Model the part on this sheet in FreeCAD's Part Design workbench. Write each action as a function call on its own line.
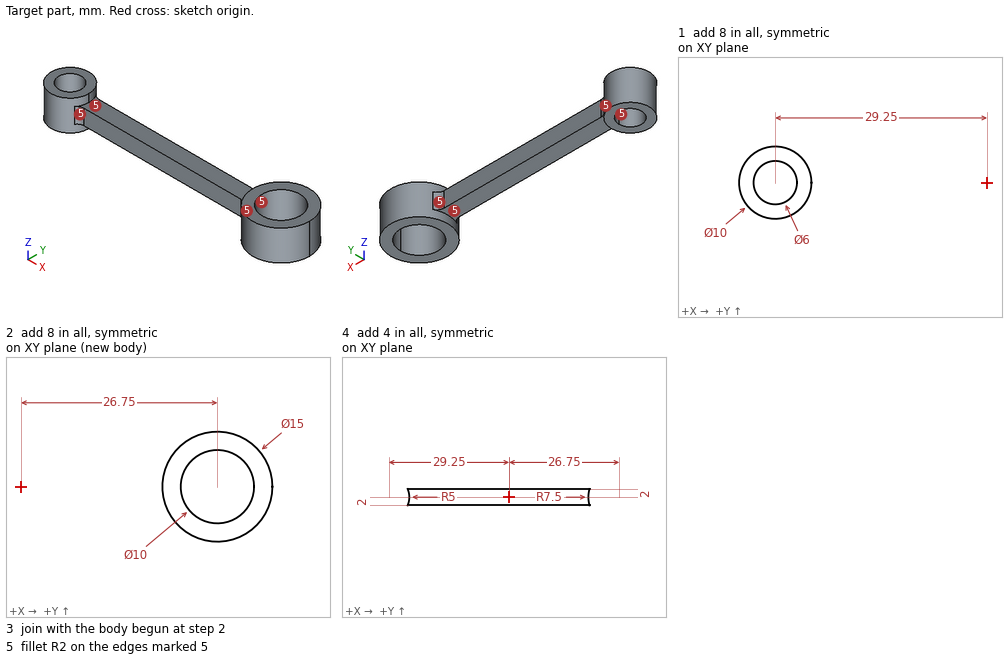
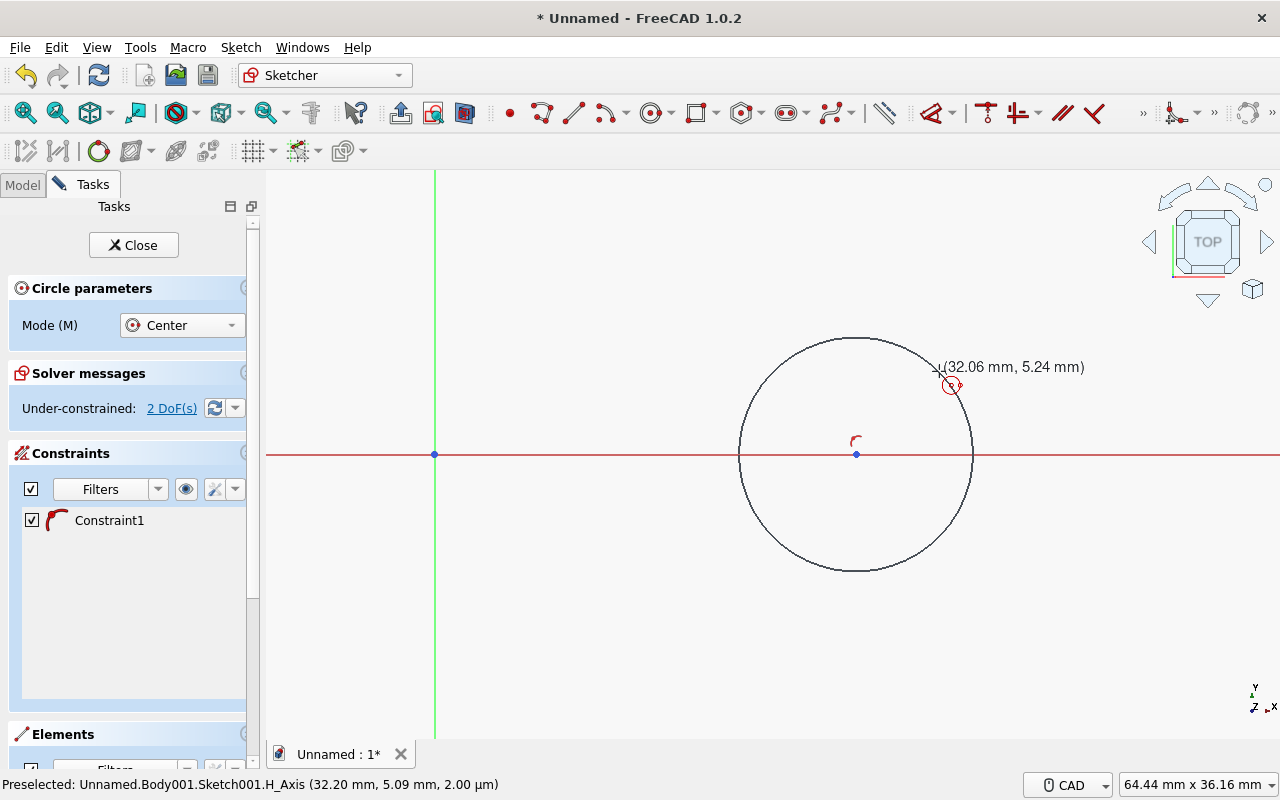
click(856, 454)
click(911, 399)
key(Escape)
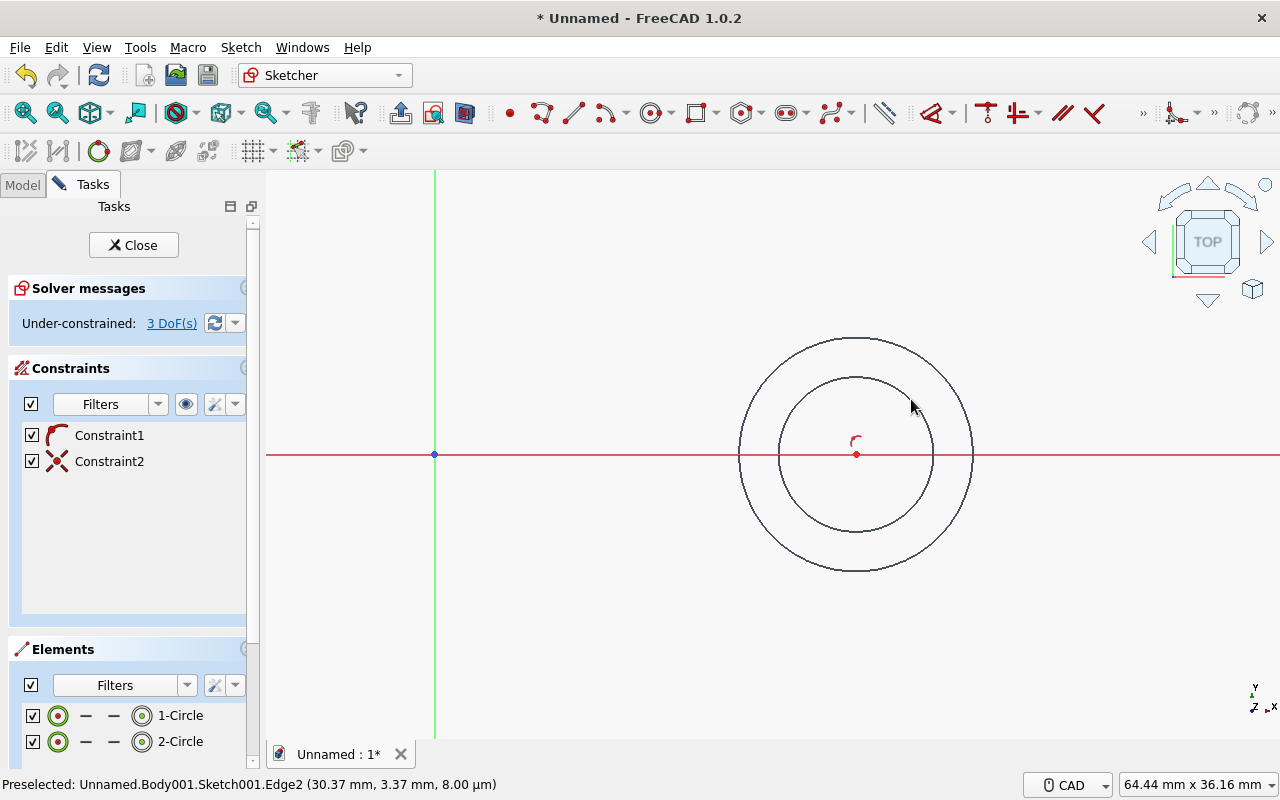
click(932, 114)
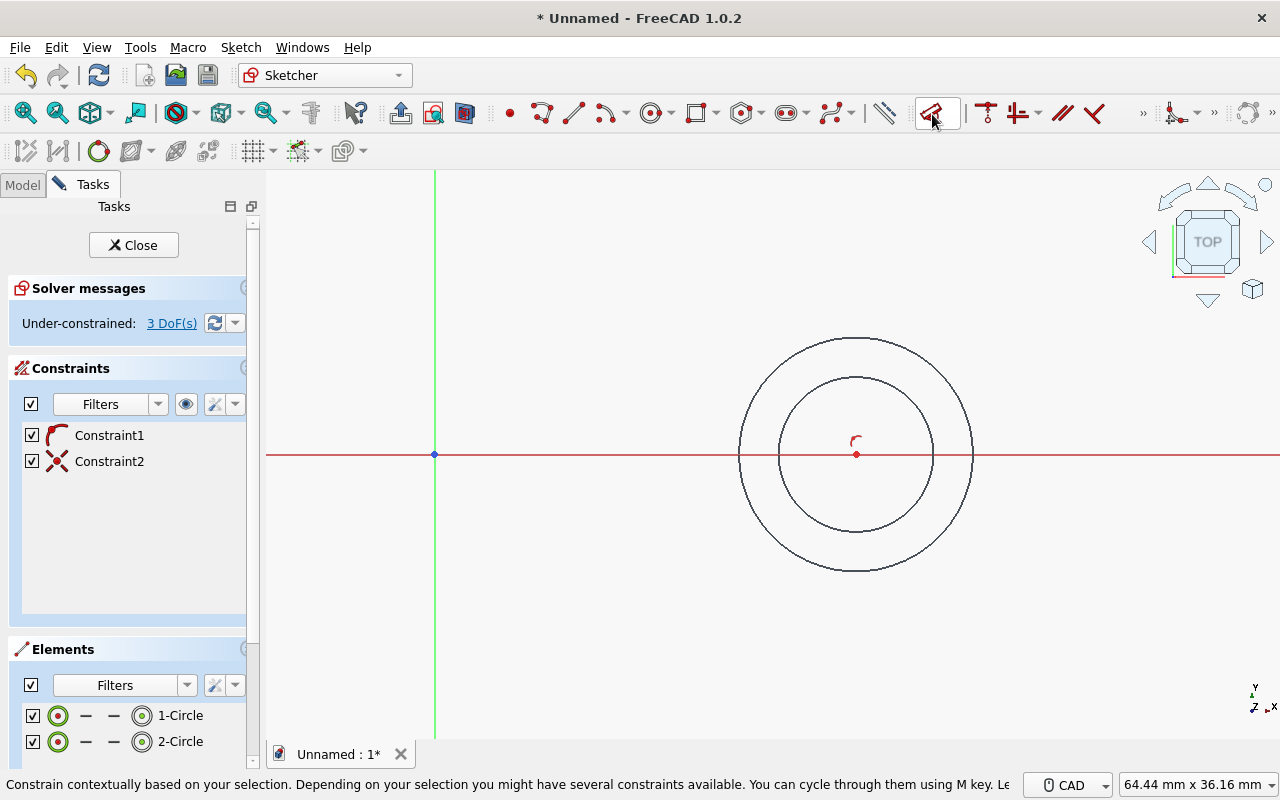
click(938, 371)
click(960, 348)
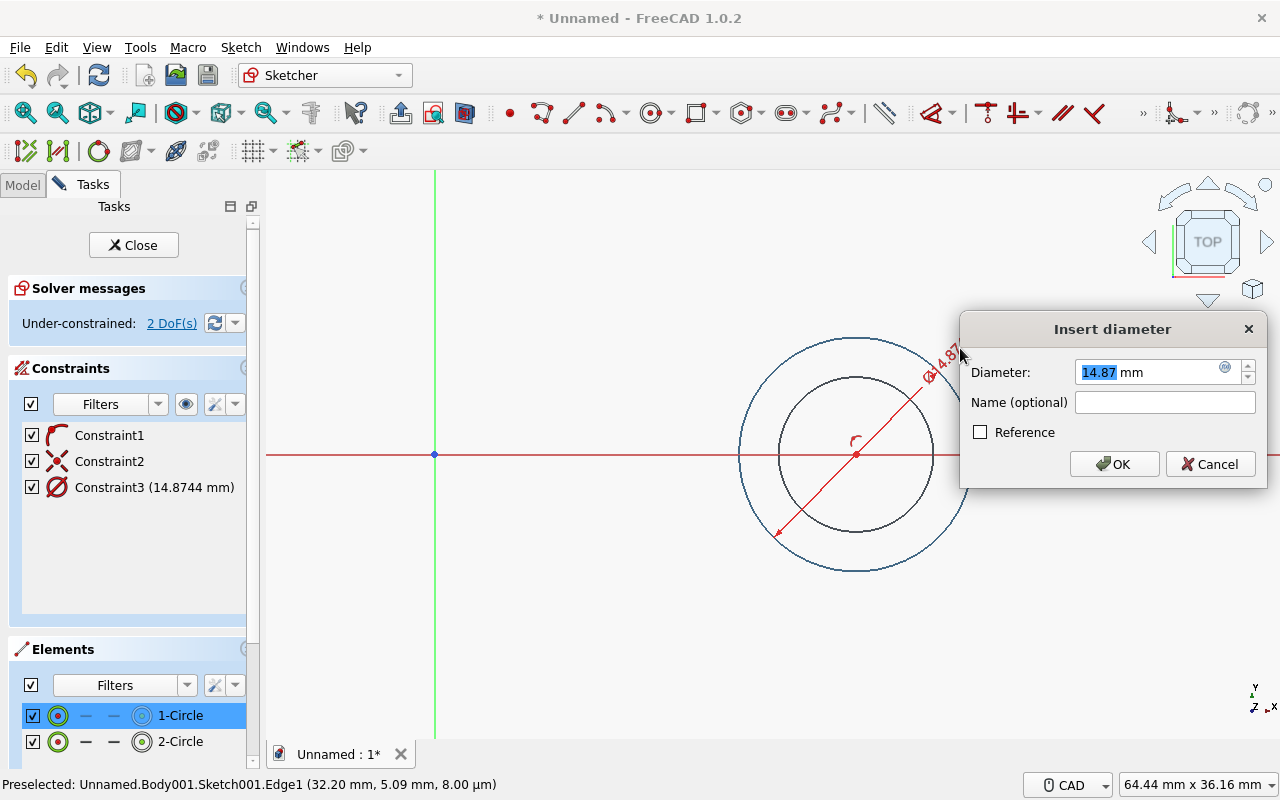
text(15)
key(Return)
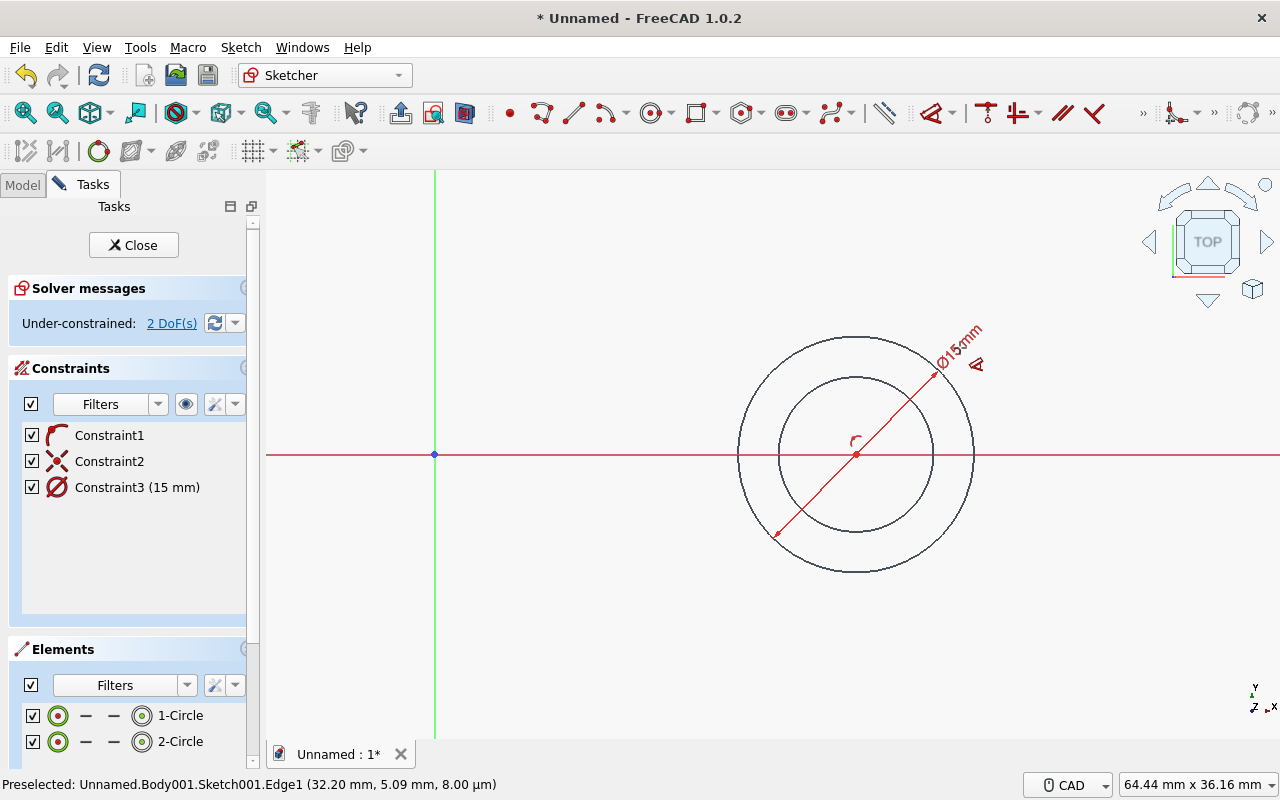
click(911, 400)
click(983, 418)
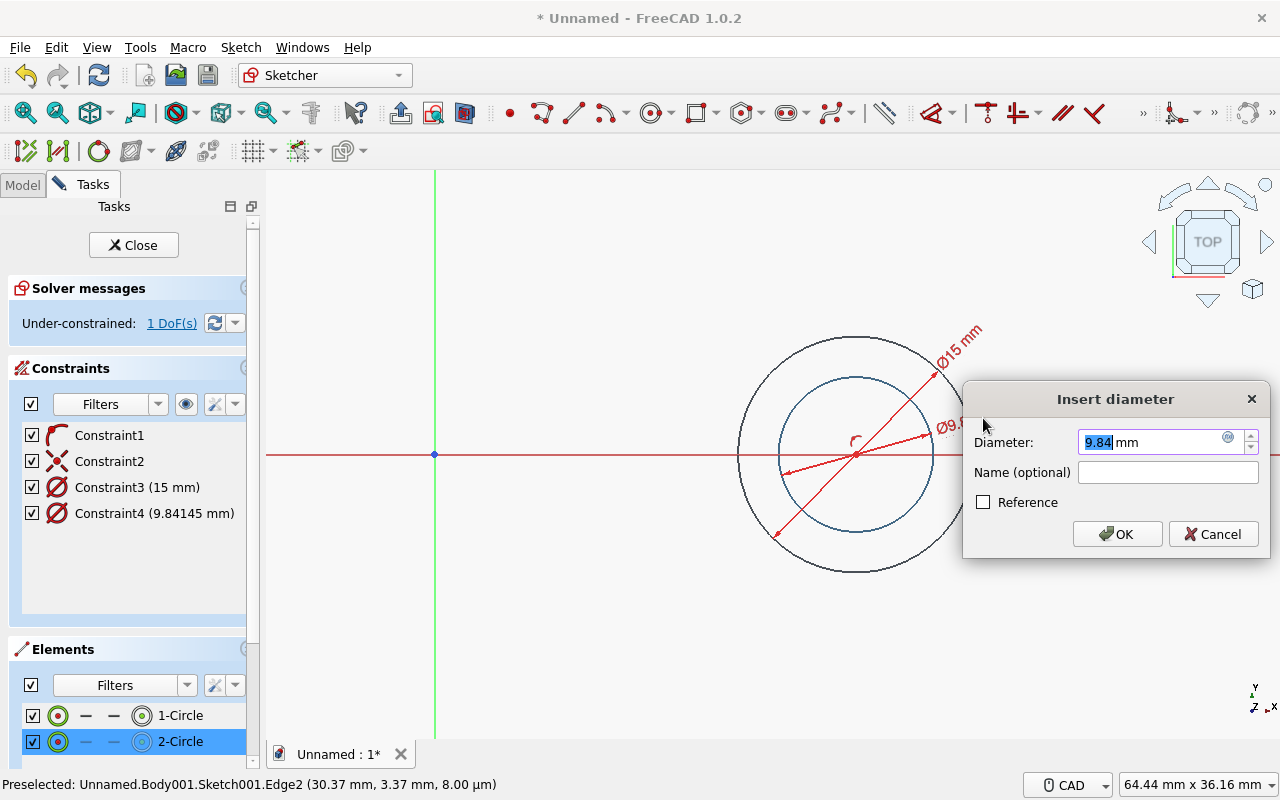
text(10)
key(Return)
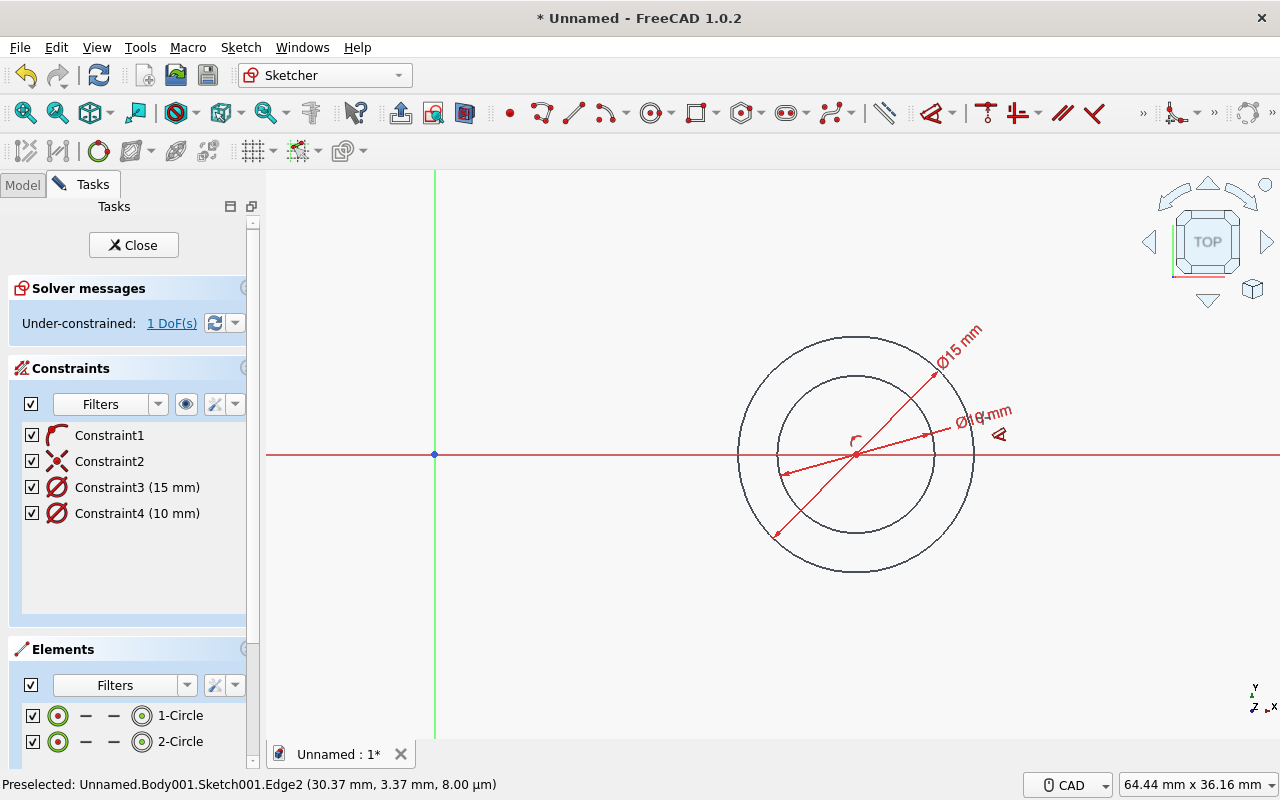
click(856, 454)
click(645, 488)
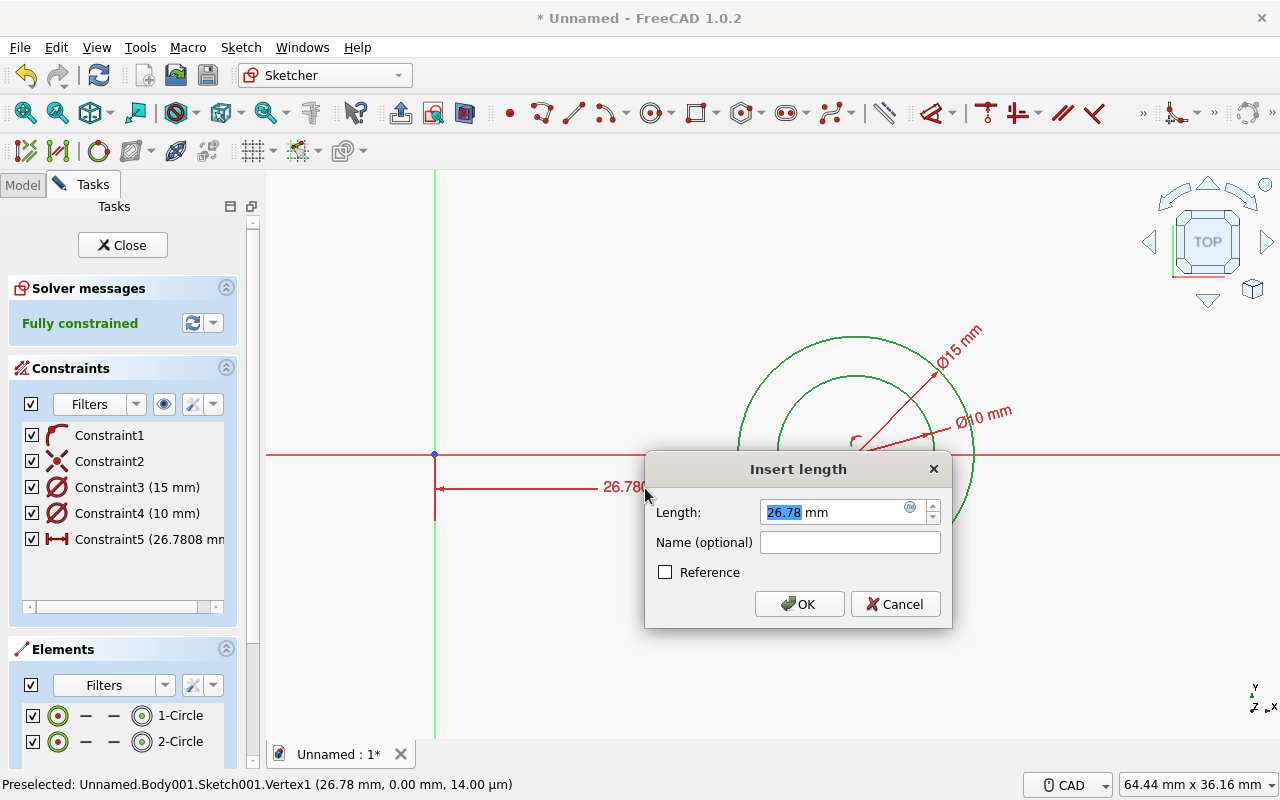
text(26.75)
key(Return)
key(Escape)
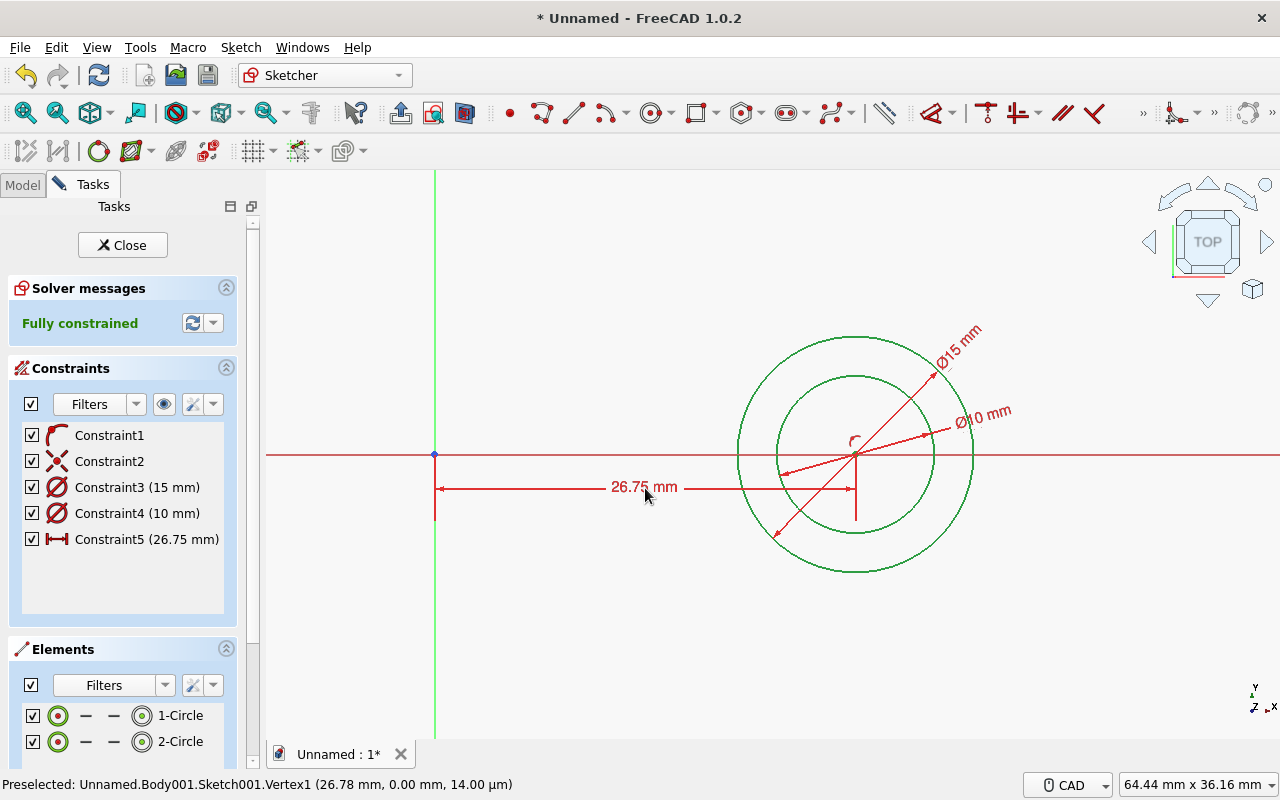
click(123, 245)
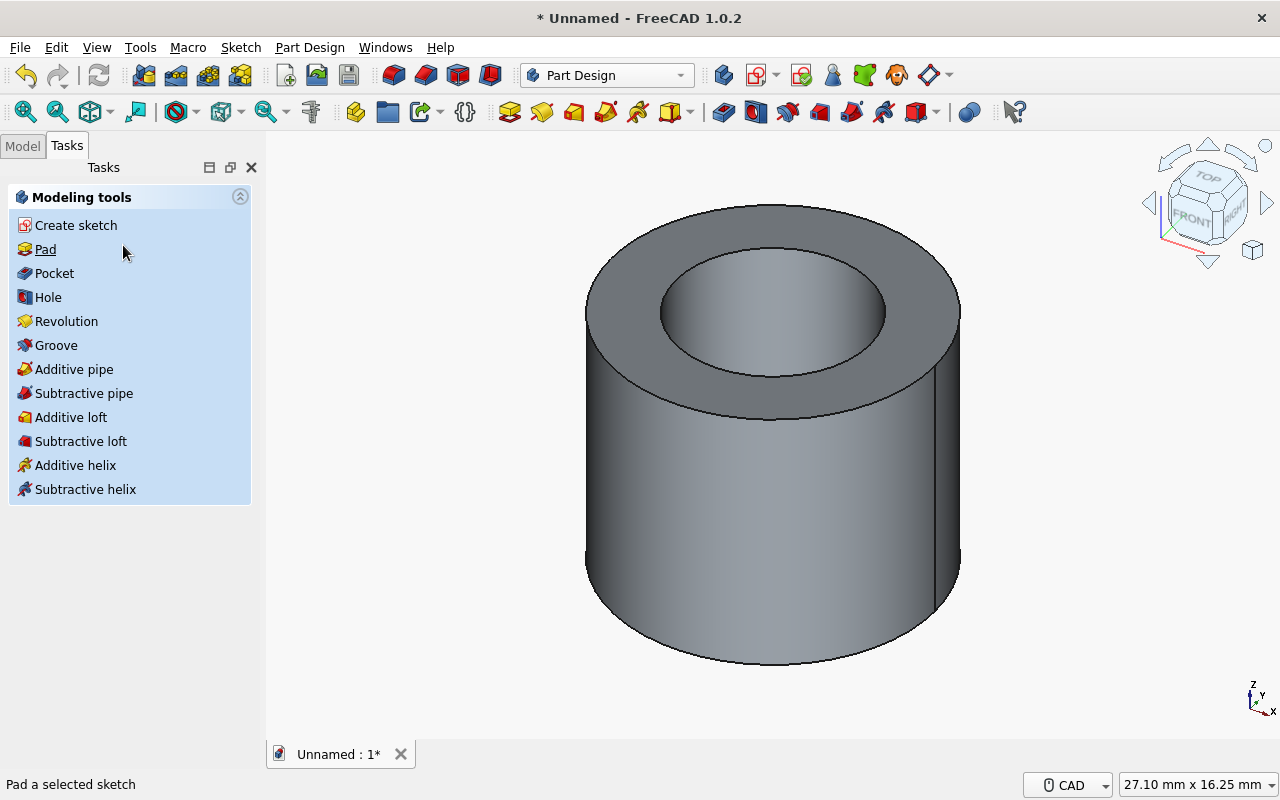
click(510, 112)